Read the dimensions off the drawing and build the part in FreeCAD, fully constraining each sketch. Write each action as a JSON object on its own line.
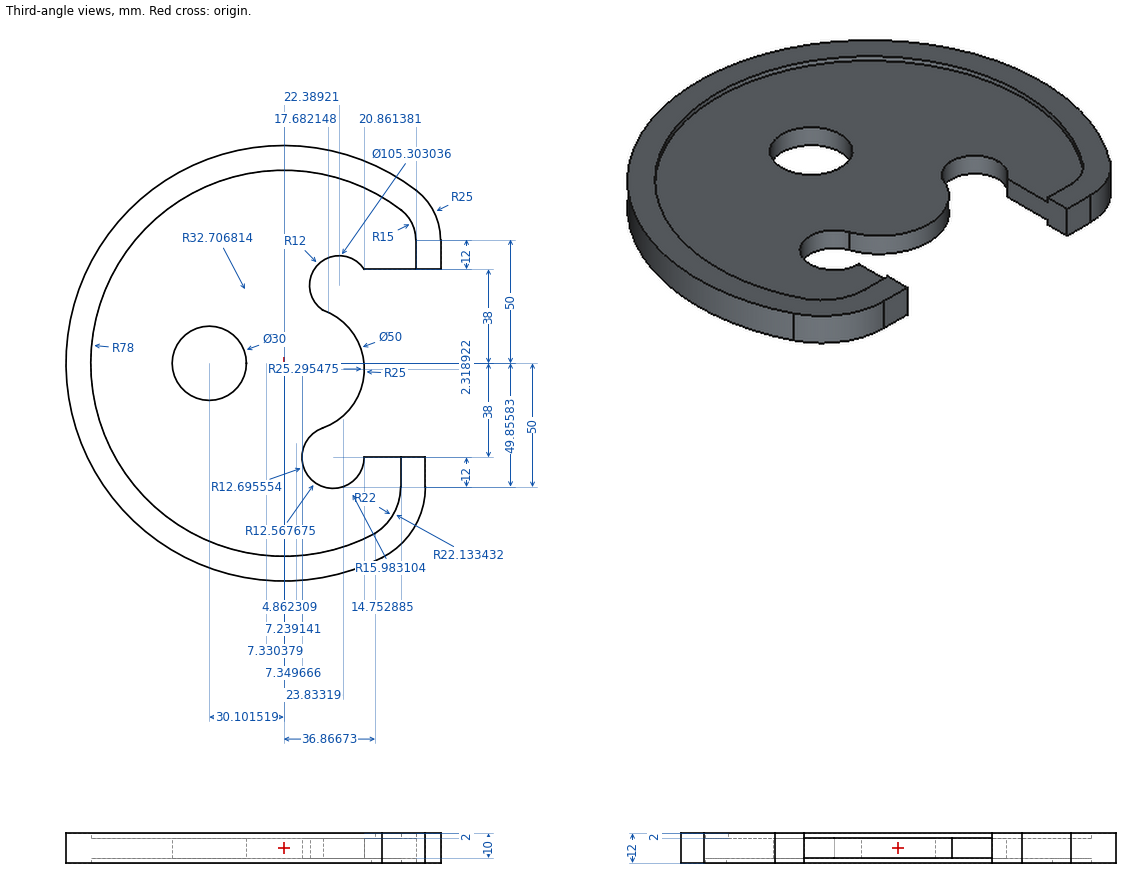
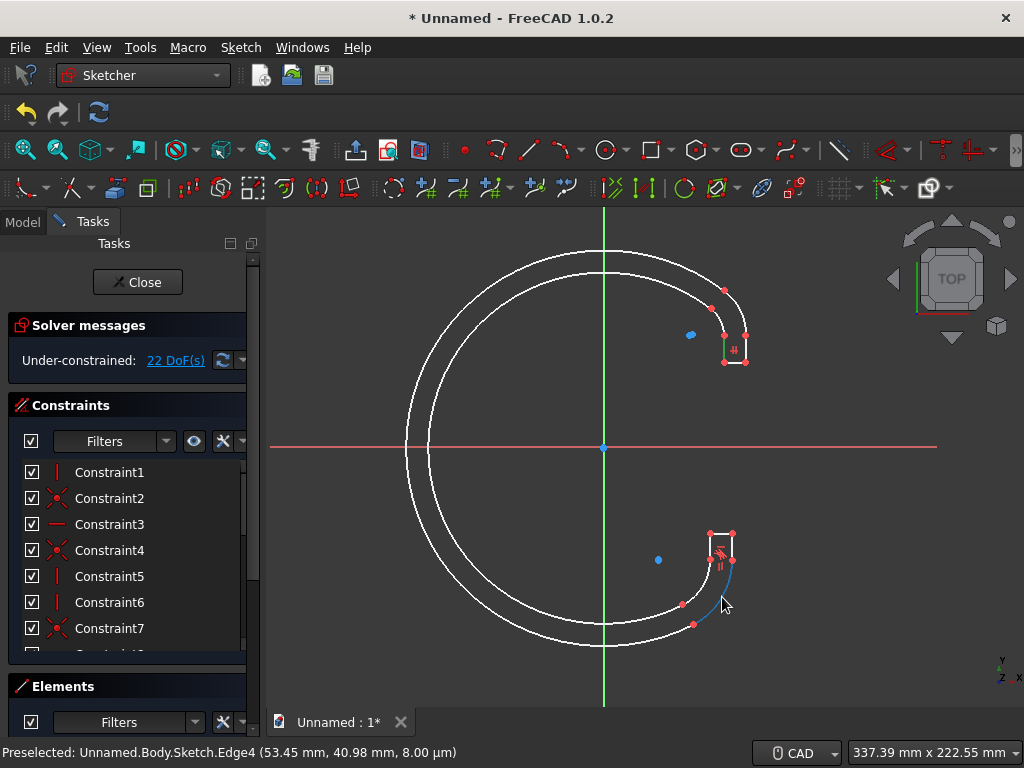
{"action": "scroll", "coordinate": [723, 327], "scroll_direction": "up", "scroll_amount": 2}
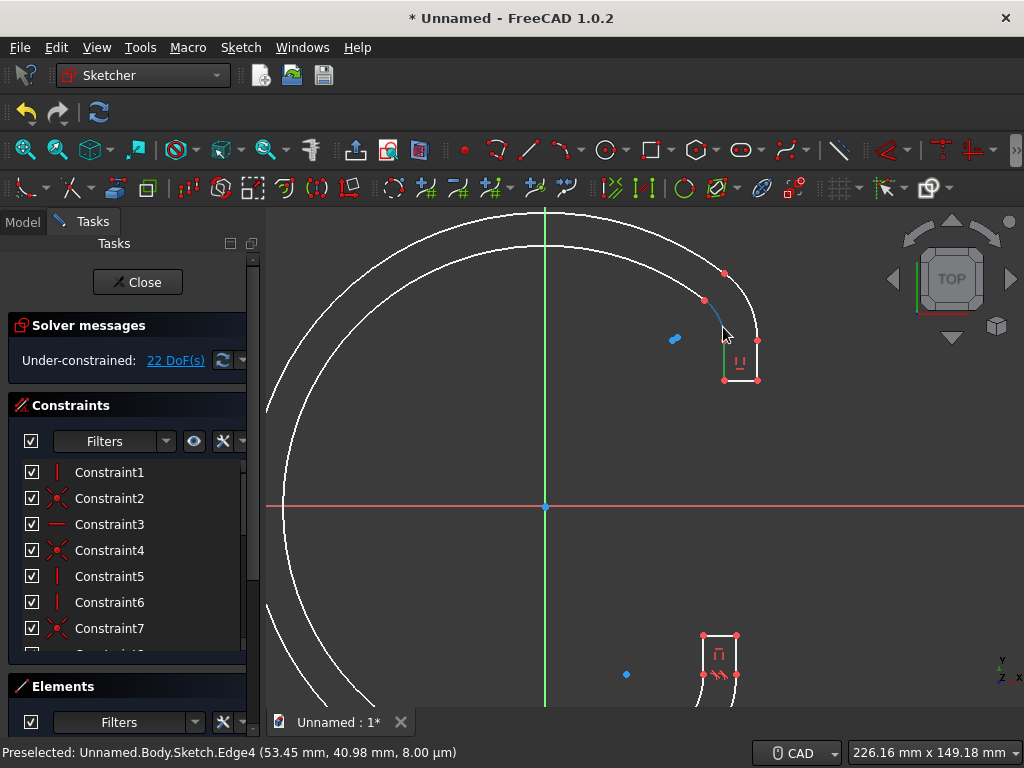
{"action": "left_click", "coordinate": [722, 327]}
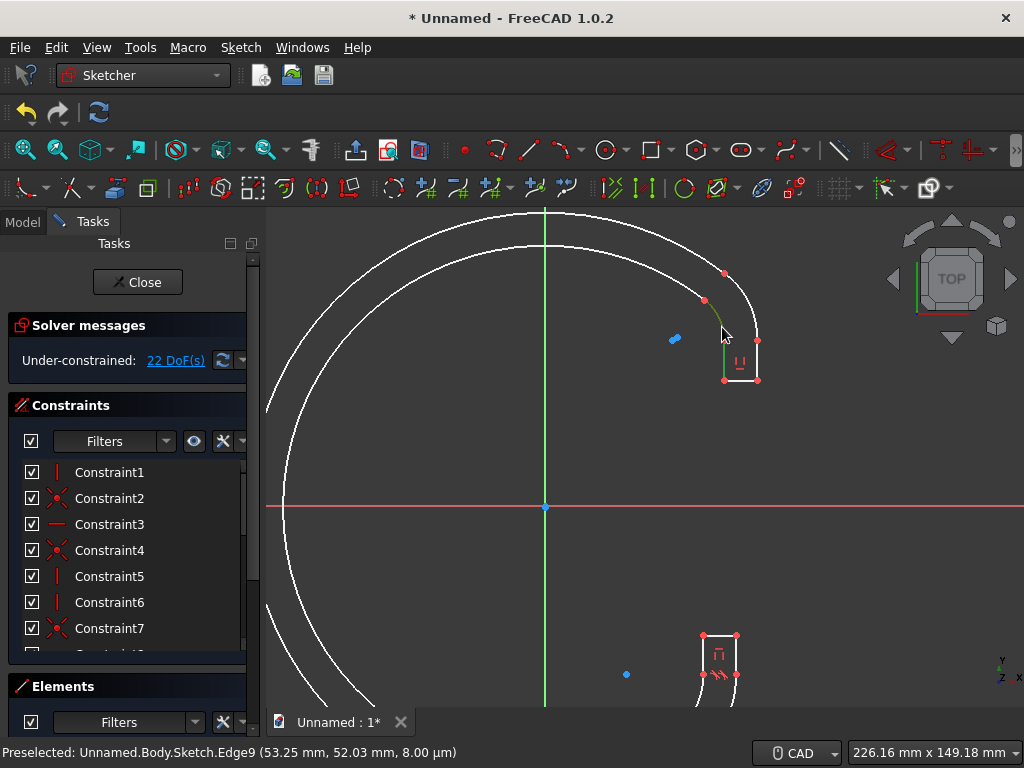
{"action": "key", "text": "t"}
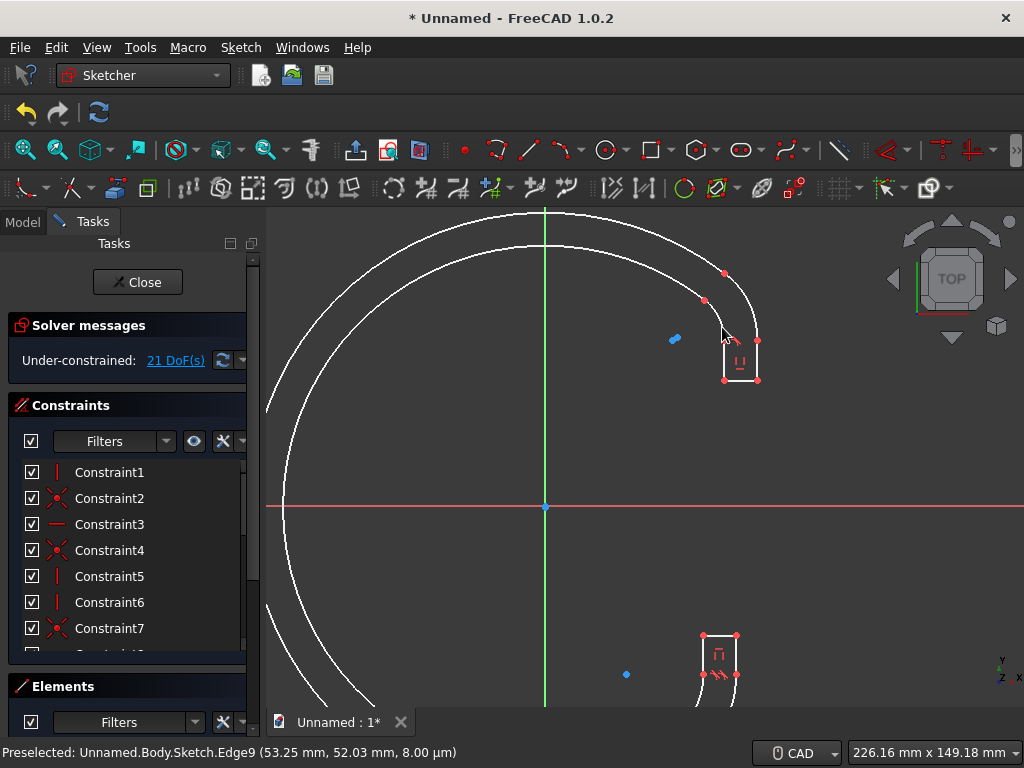
{"action": "left_click", "coordinate": [757, 369]}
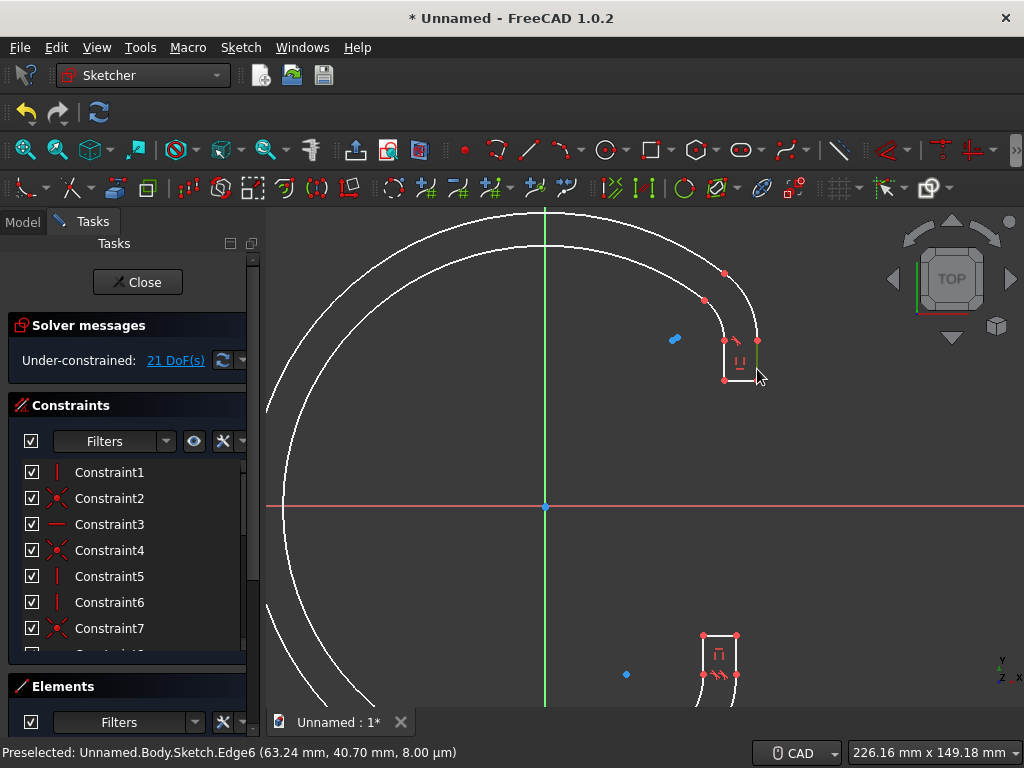
{"action": "left_click", "coordinate": [754, 317]}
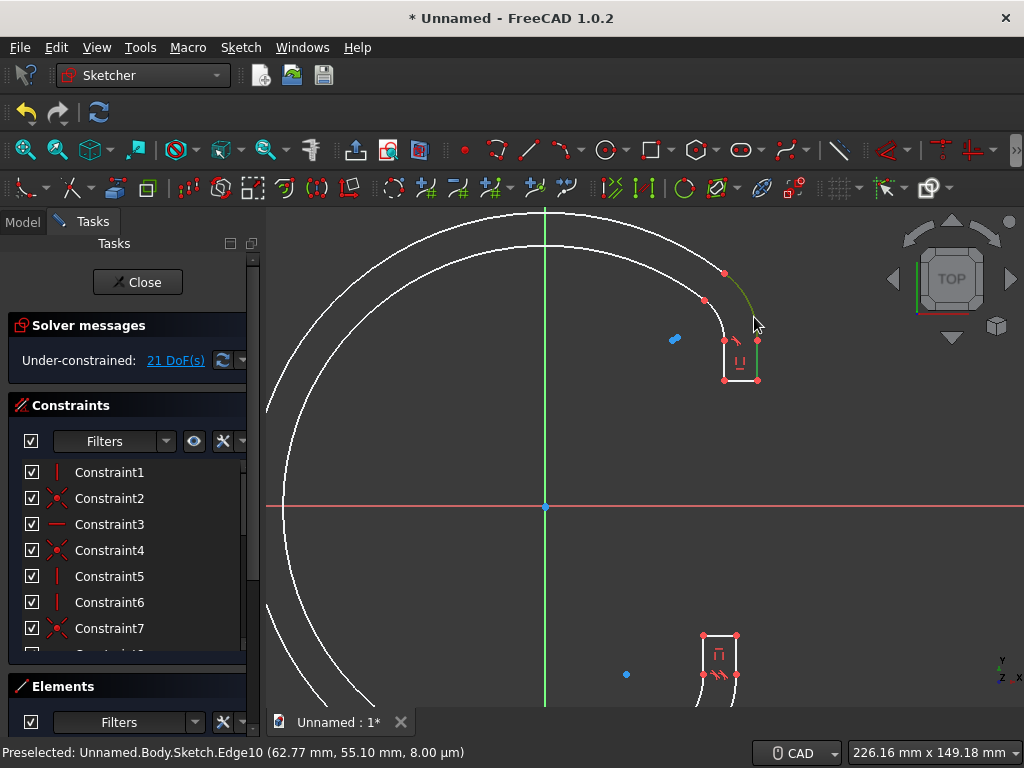
{"action": "key", "text": "t"}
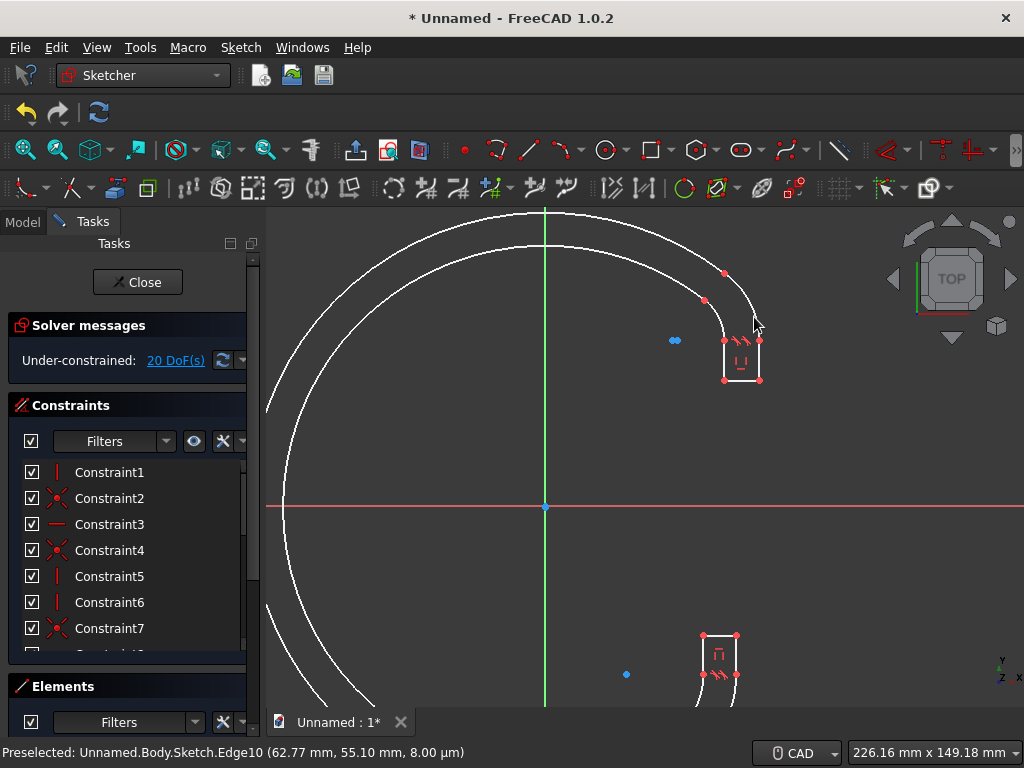
{"action": "scroll", "coordinate": [723, 327], "scroll_direction": "down", "scroll_amount": 2}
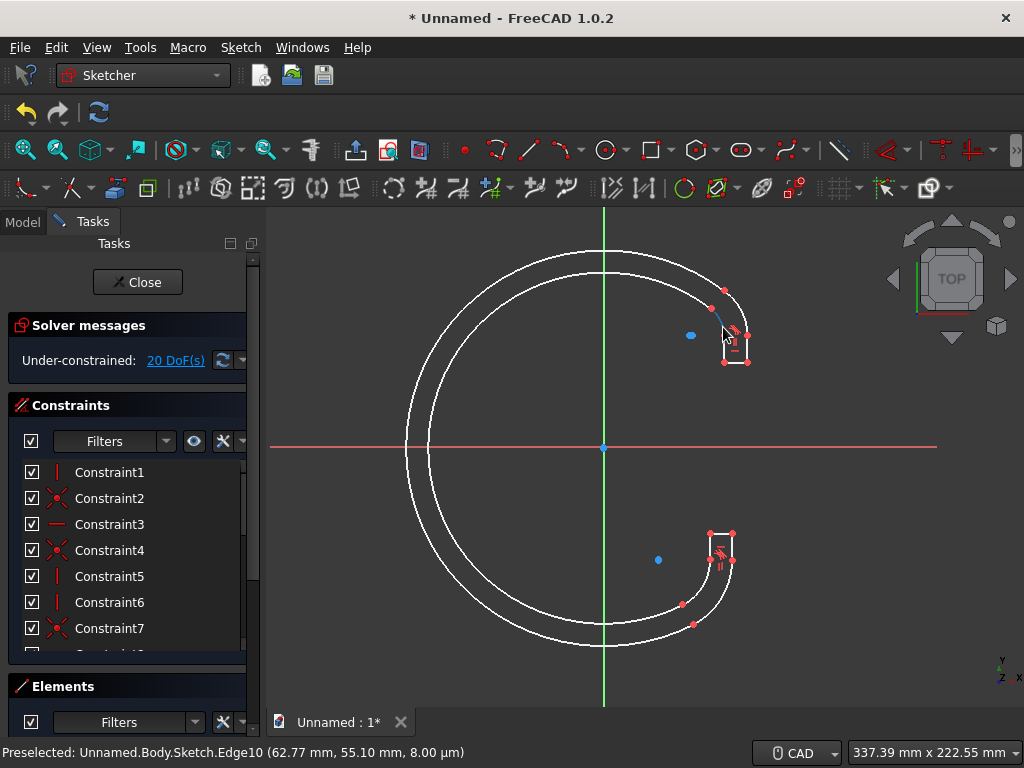
{"action": "left_click", "coordinate": [696, 595]}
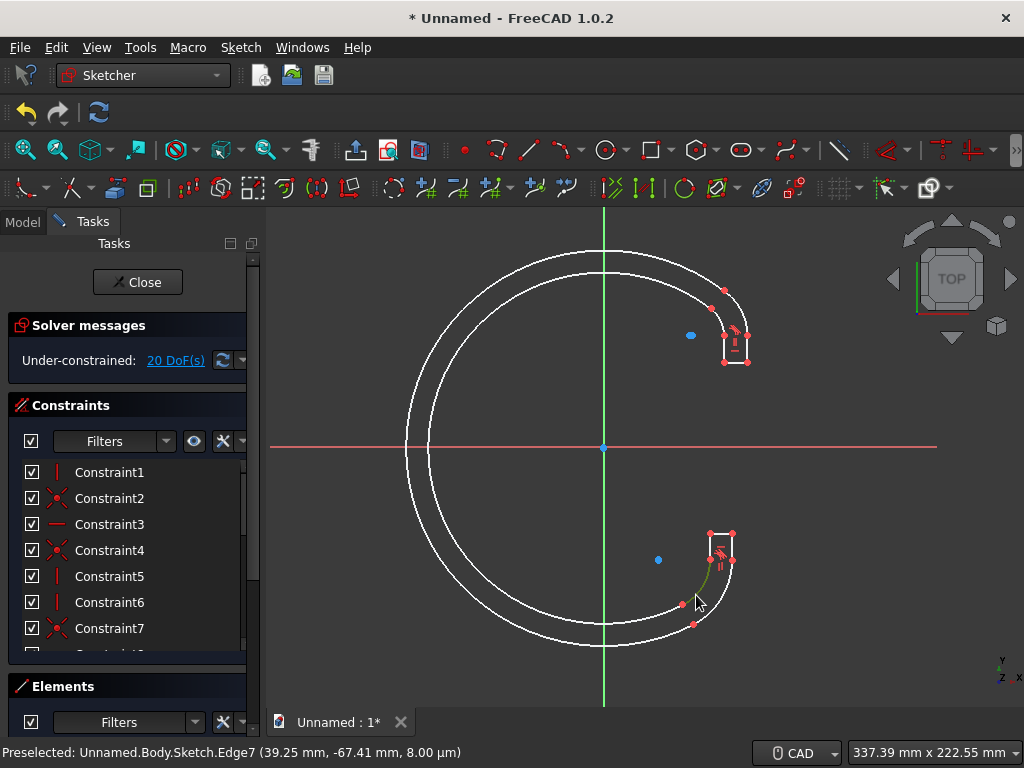
{"action": "left_click", "coordinate": [501, 306]}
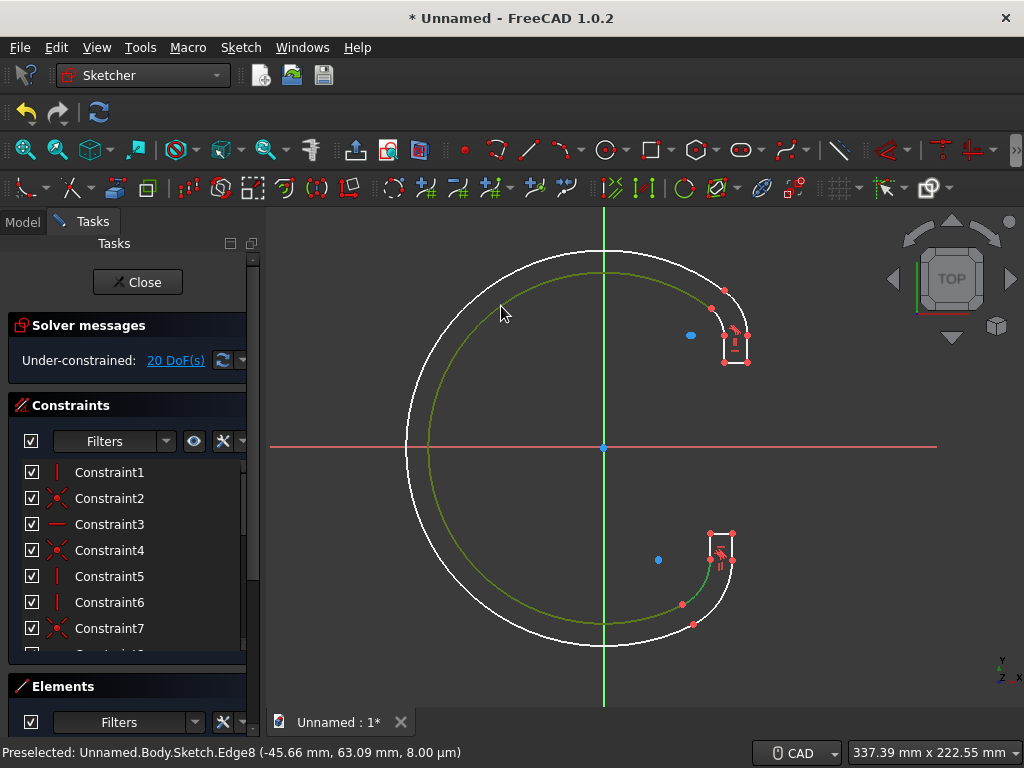
{"action": "key", "text": "t"}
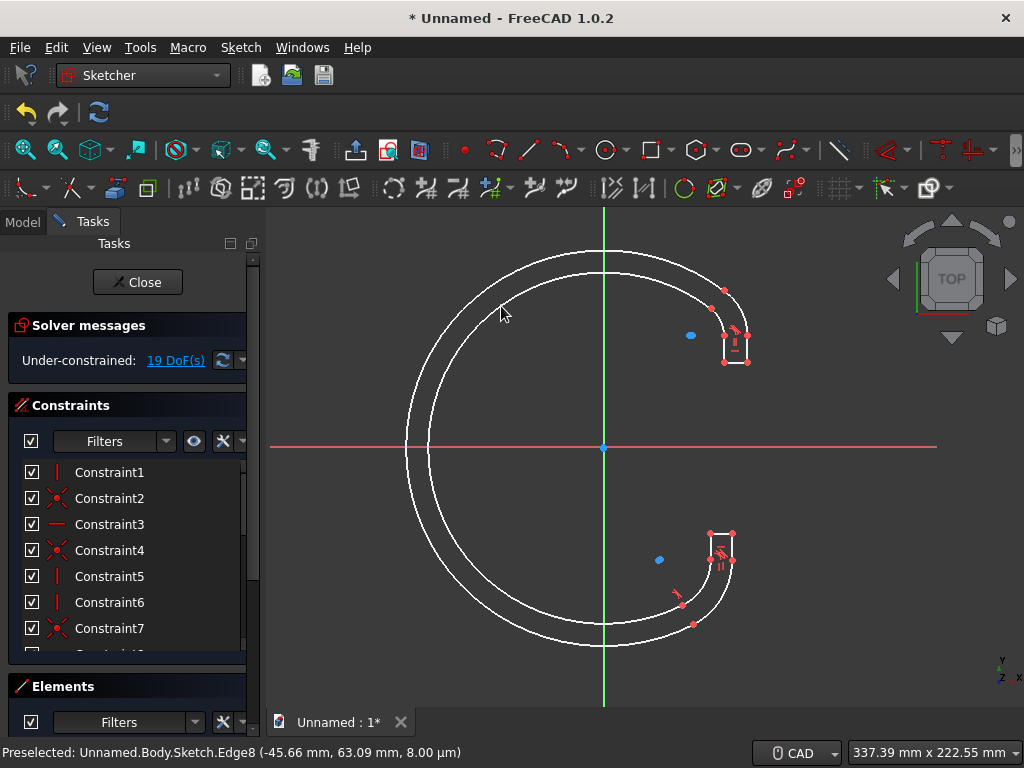
{"action": "left_click", "coordinate": [501, 306]}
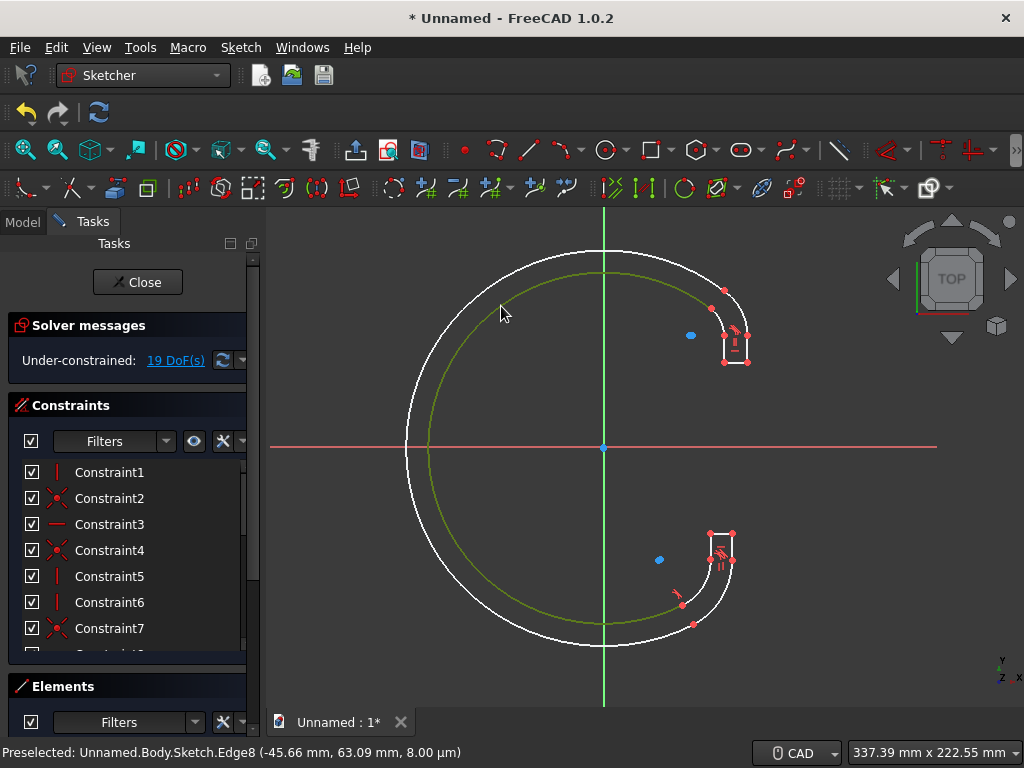
{"action": "scroll", "coordinate": [723, 327], "scroll_direction": "up", "scroll_amount": 2}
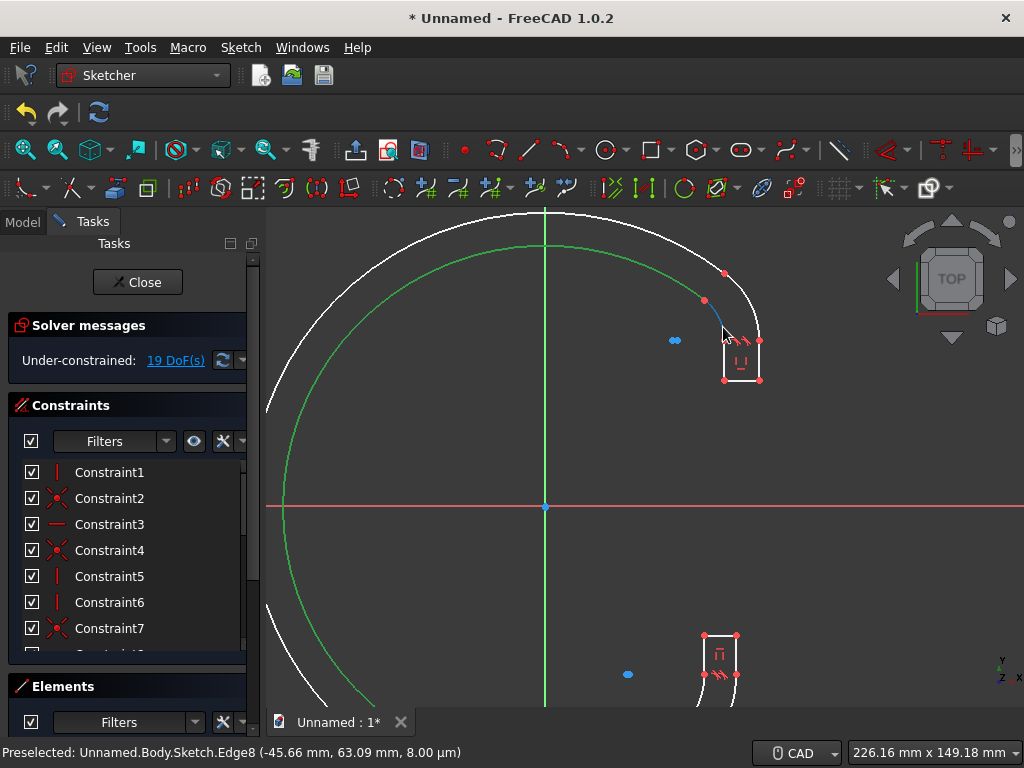
{"action": "left_click", "coordinate": [722, 327]}